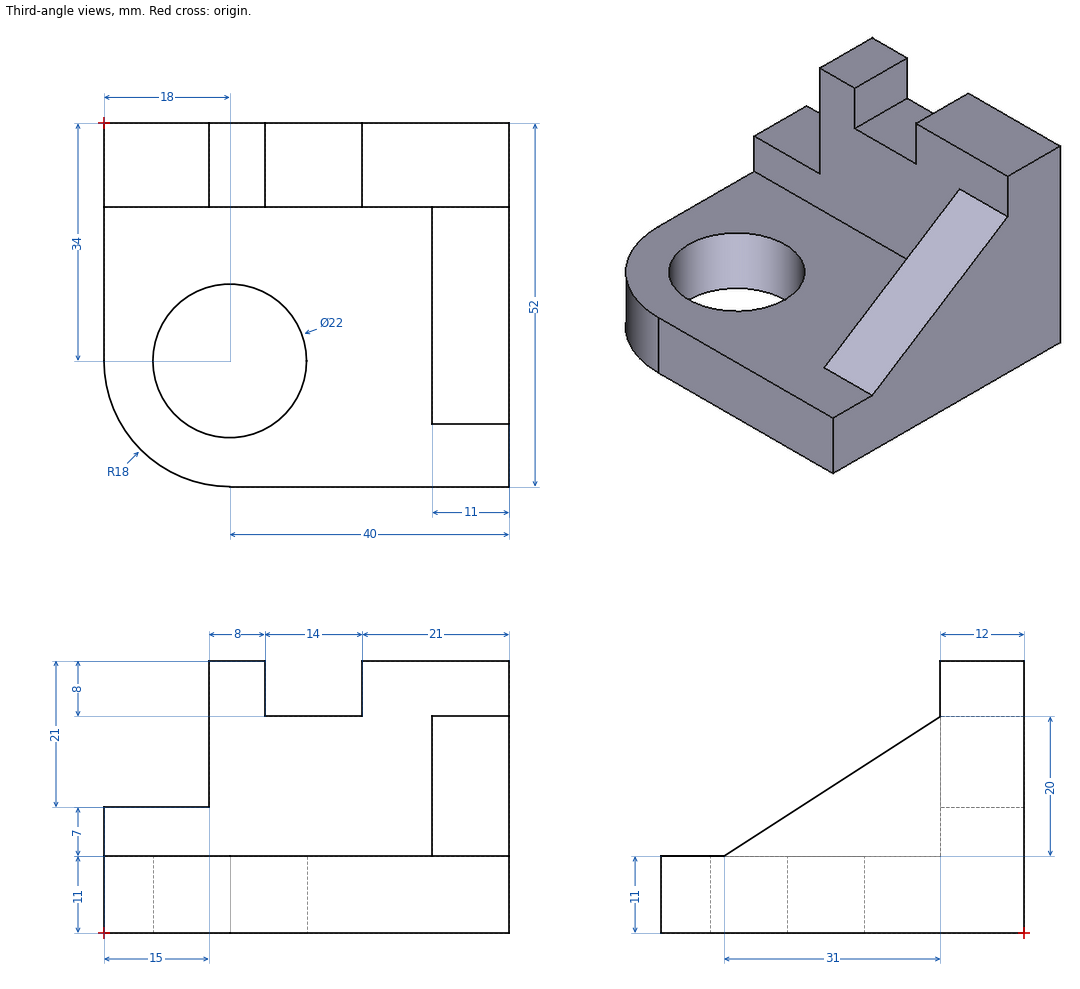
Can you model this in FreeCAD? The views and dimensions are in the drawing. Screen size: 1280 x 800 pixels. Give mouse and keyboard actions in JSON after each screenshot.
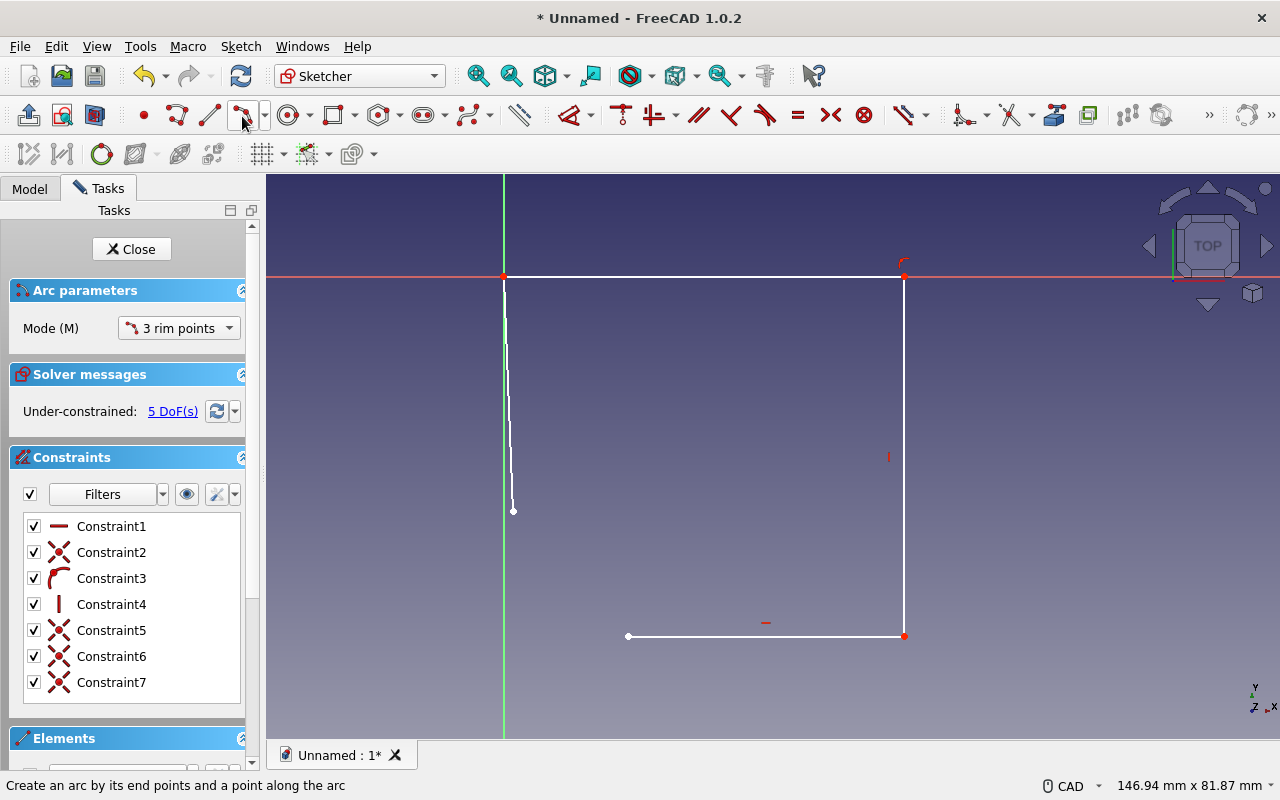
{"action": "left_click", "coordinate": [513, 512]}
{"action": "left_click", "coordinate": [628, 637]}
{"action": "left_click", "coordinate": [540, 599]}
{"action": "key", "text": "Escape"}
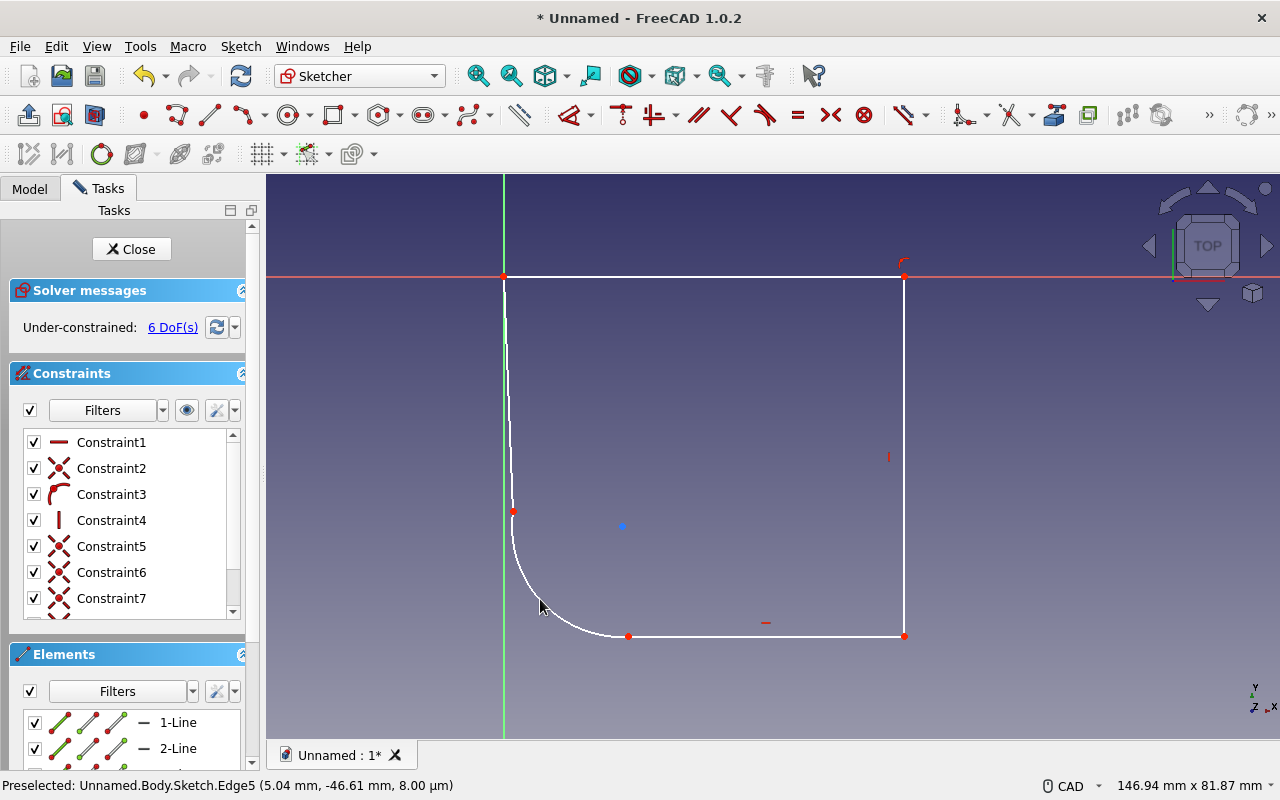
{"action": "left_click", "coordinate": [711, 637]}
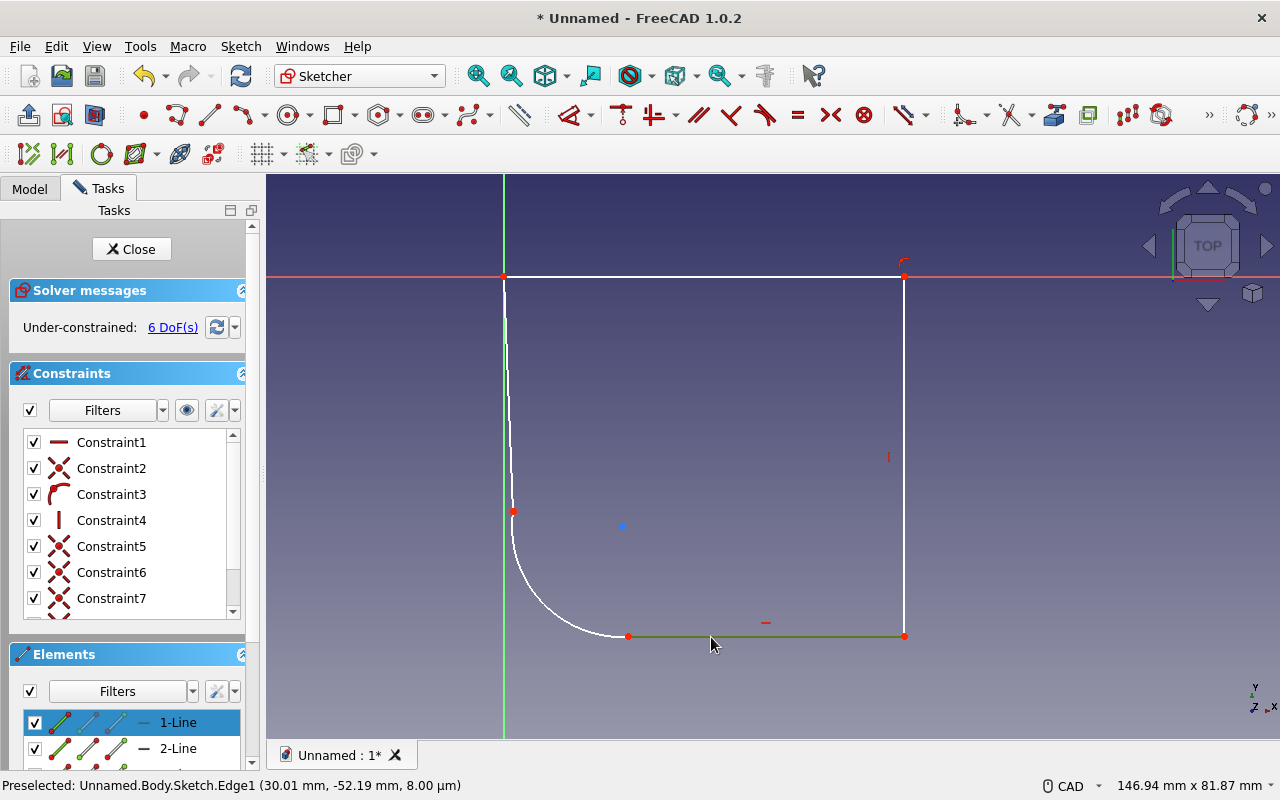
{"action": "left_click", "coordinate": [521, 569]}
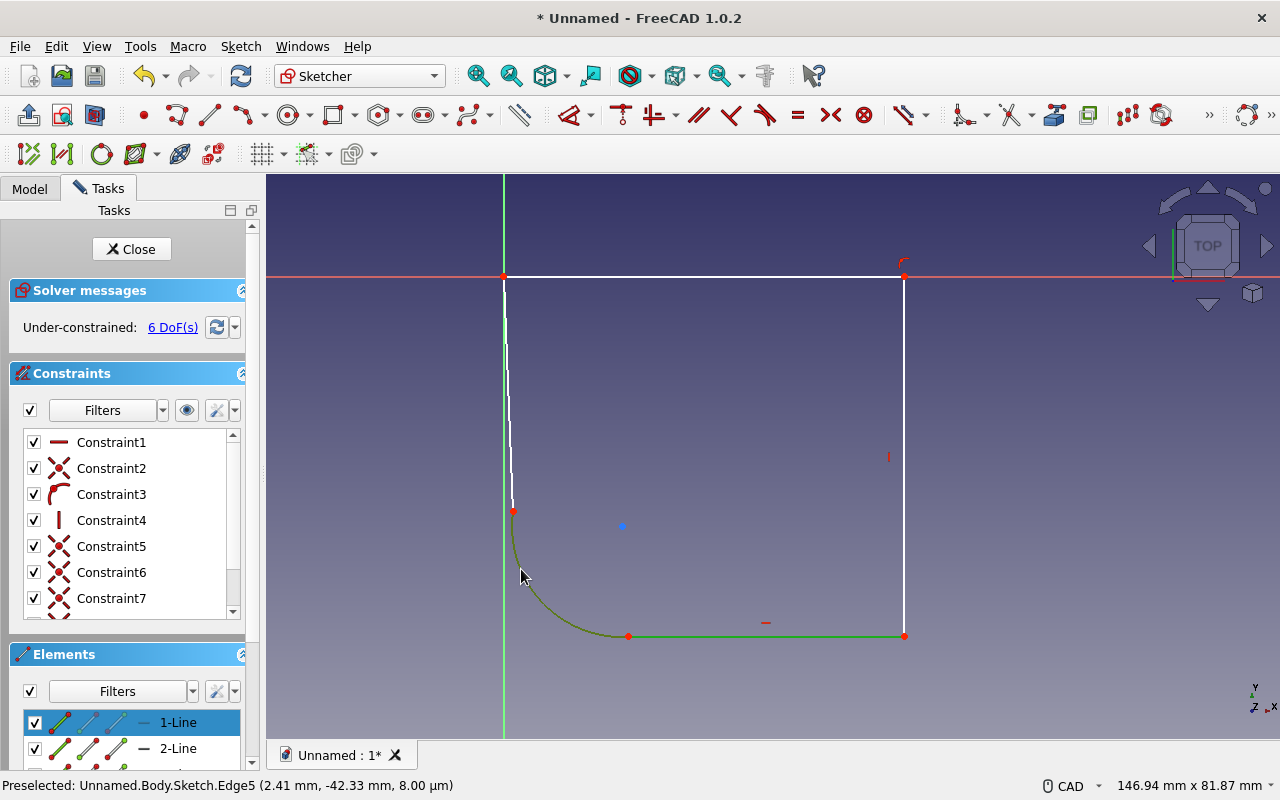
{"action": "left_click", "coordinate": [765, 116]}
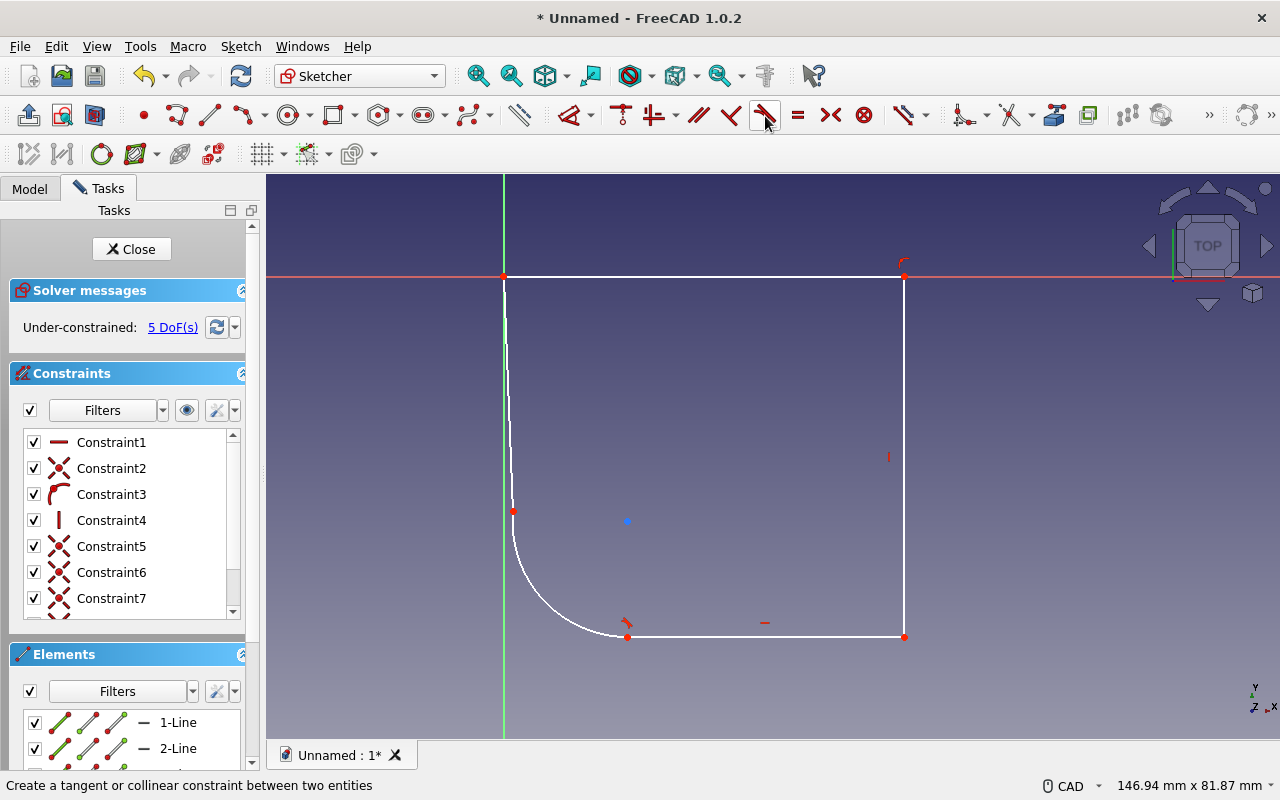
{"action": "left_click", "coordinate": [507, 347]}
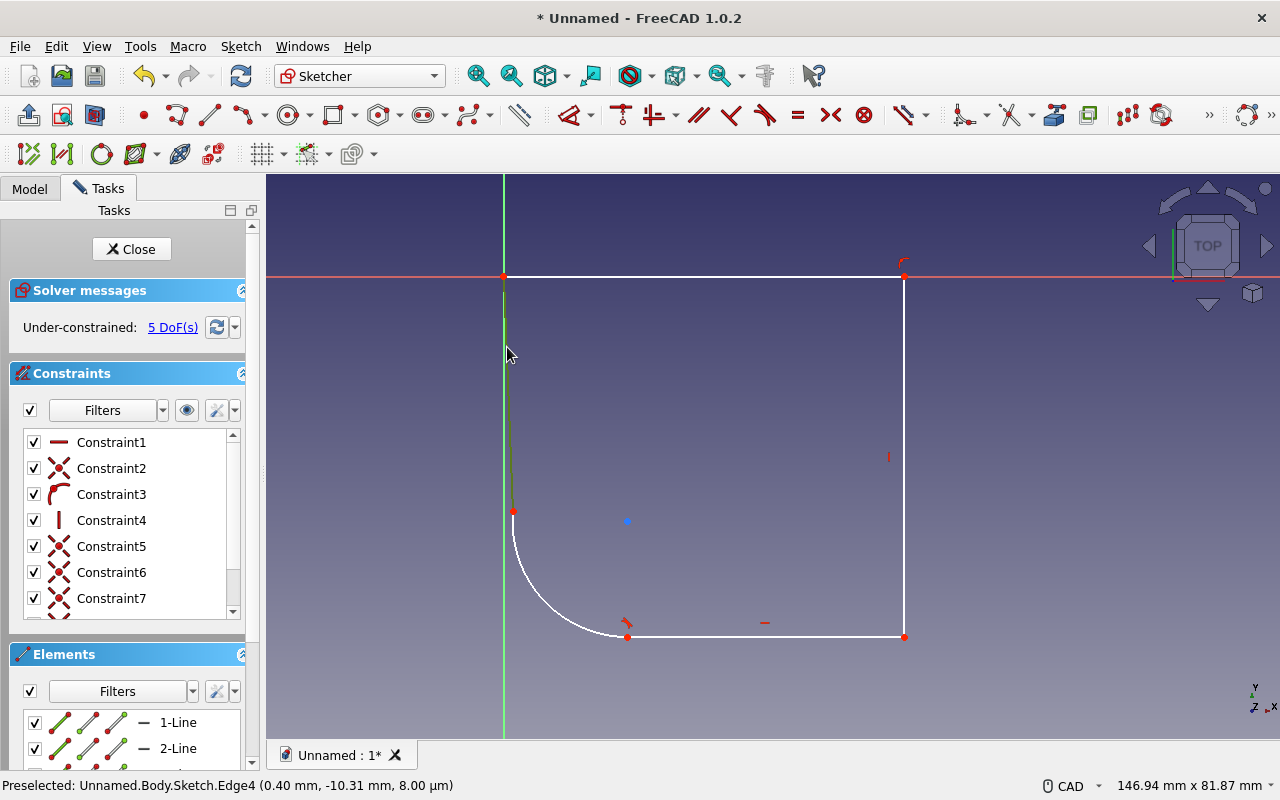
{"action": "left_click", "coordinate": [522, 568]}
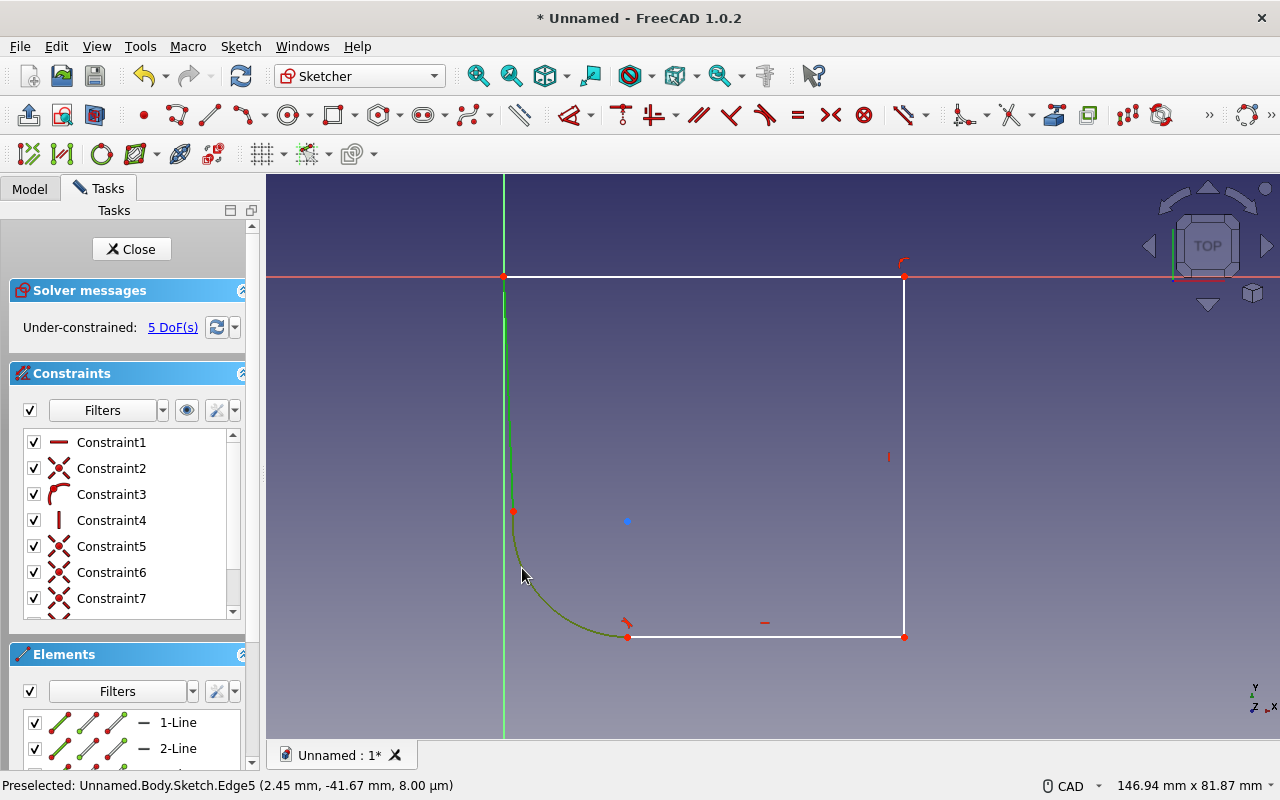
{"action": "left_click", "coordinate": [765, 116]}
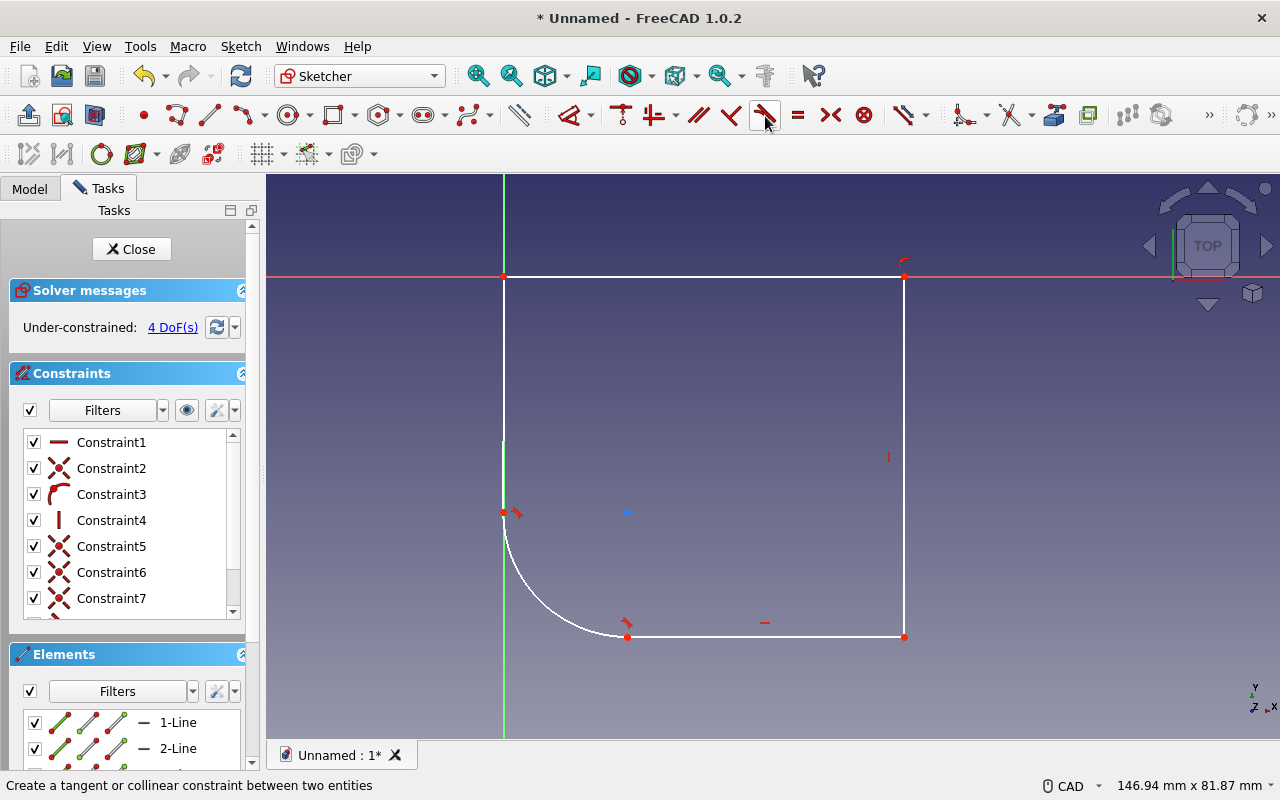
{"action": "left_click", "coordinate": [504, 347]}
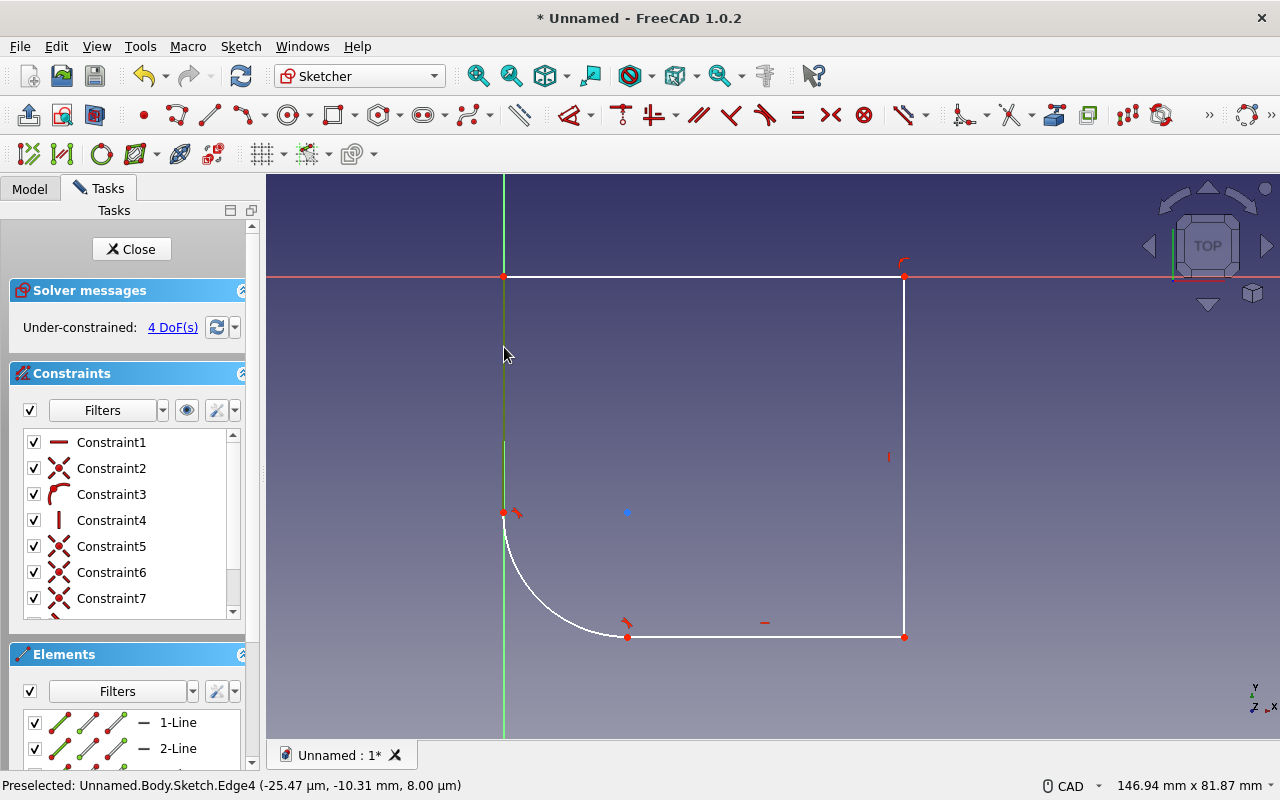
{"action": "key", "text": "v"}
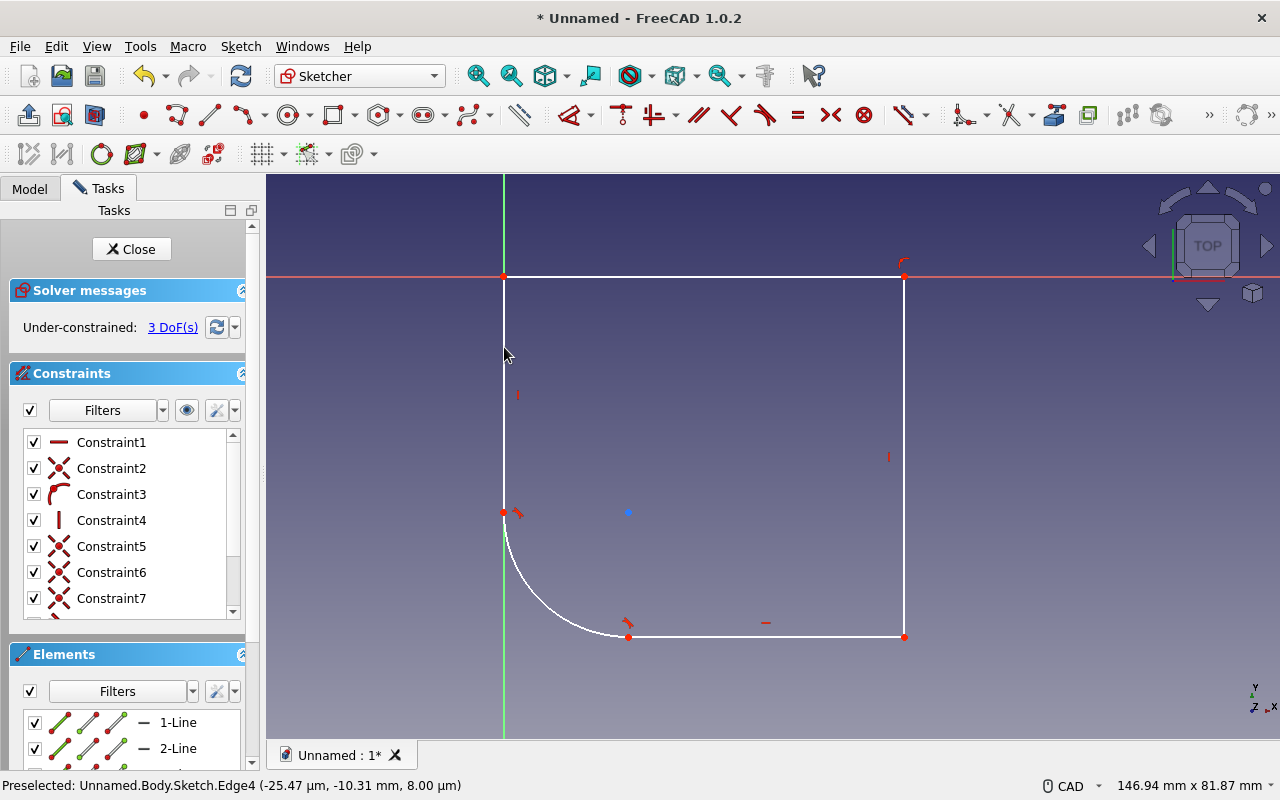
{"action": "left_click", "coordinate": [568, 116]}